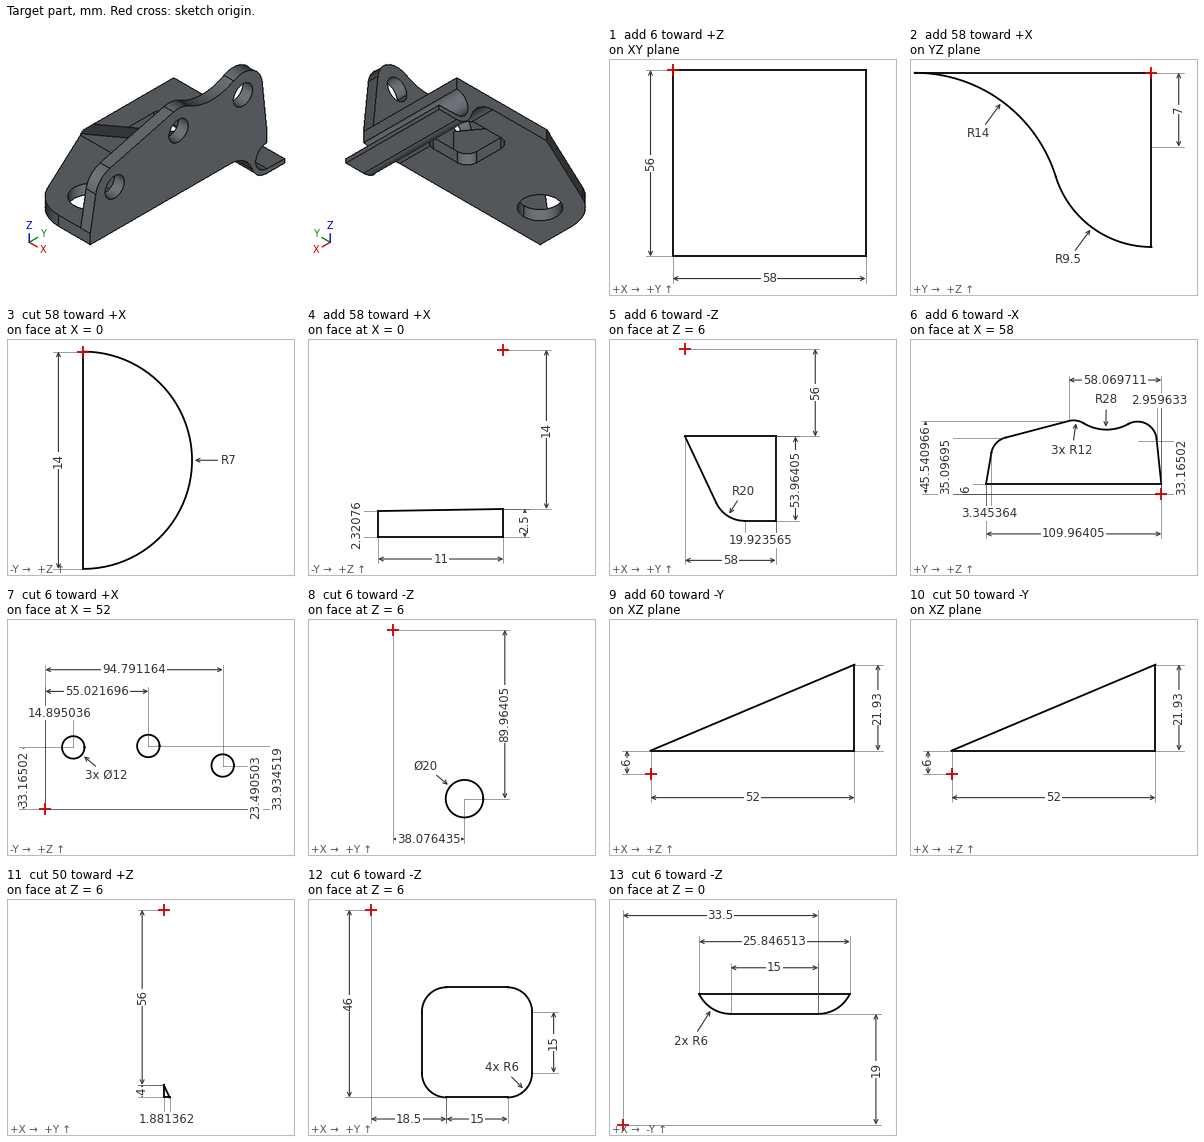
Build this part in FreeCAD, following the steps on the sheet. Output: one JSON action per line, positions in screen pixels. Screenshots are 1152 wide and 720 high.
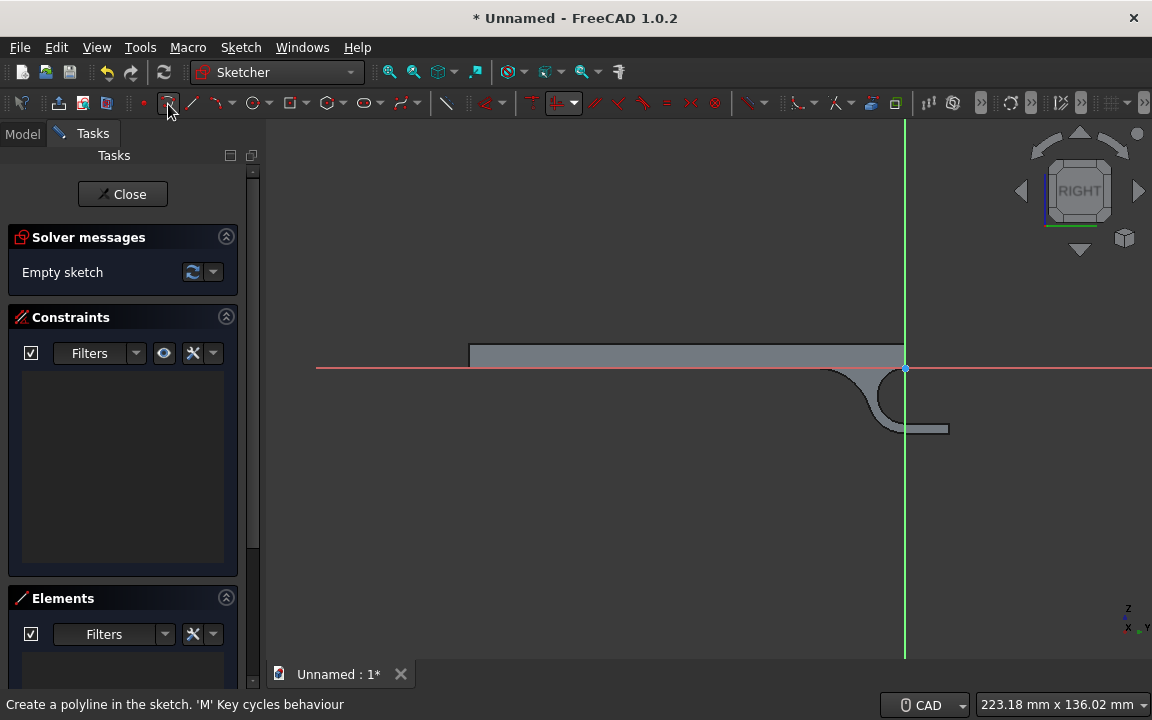
{"action": "left_click", "coordinate": [482, 267]}
{"action": "left_click", "coordinate": [469, 344]}
{"action": "left_click", "coordinate": [905, 344]}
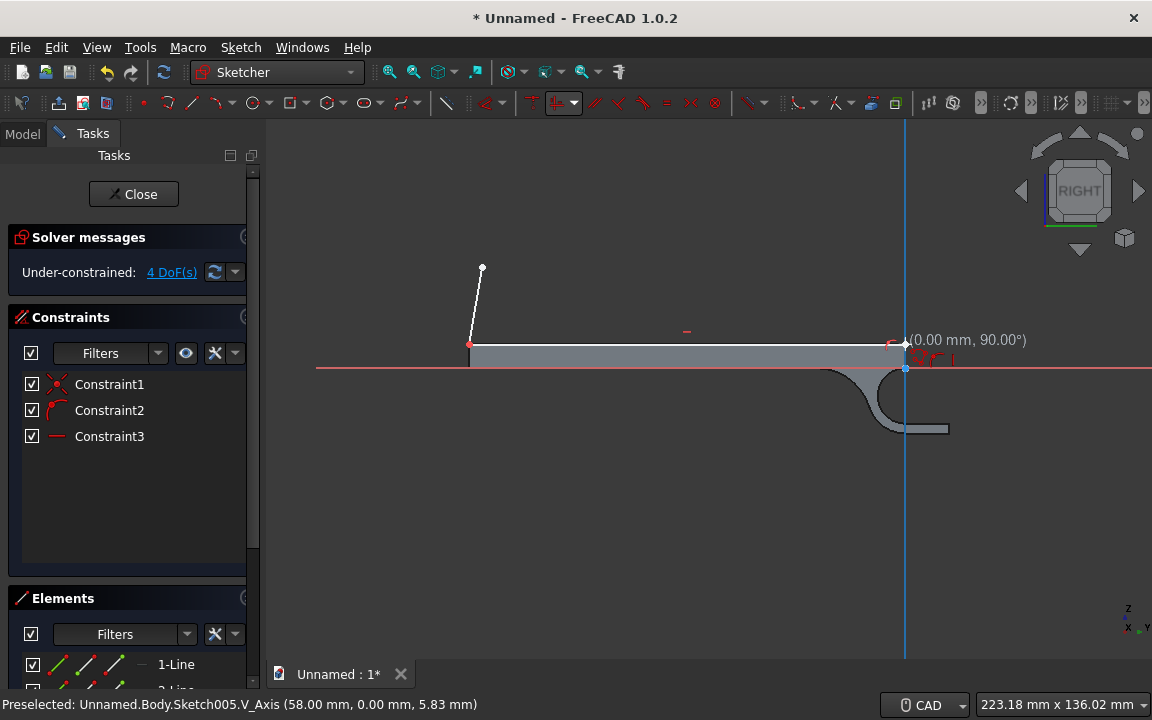
{"action": "scroll", "coordinate": [894, 232], "scroll_direction": "up", "scroll_amount": 2}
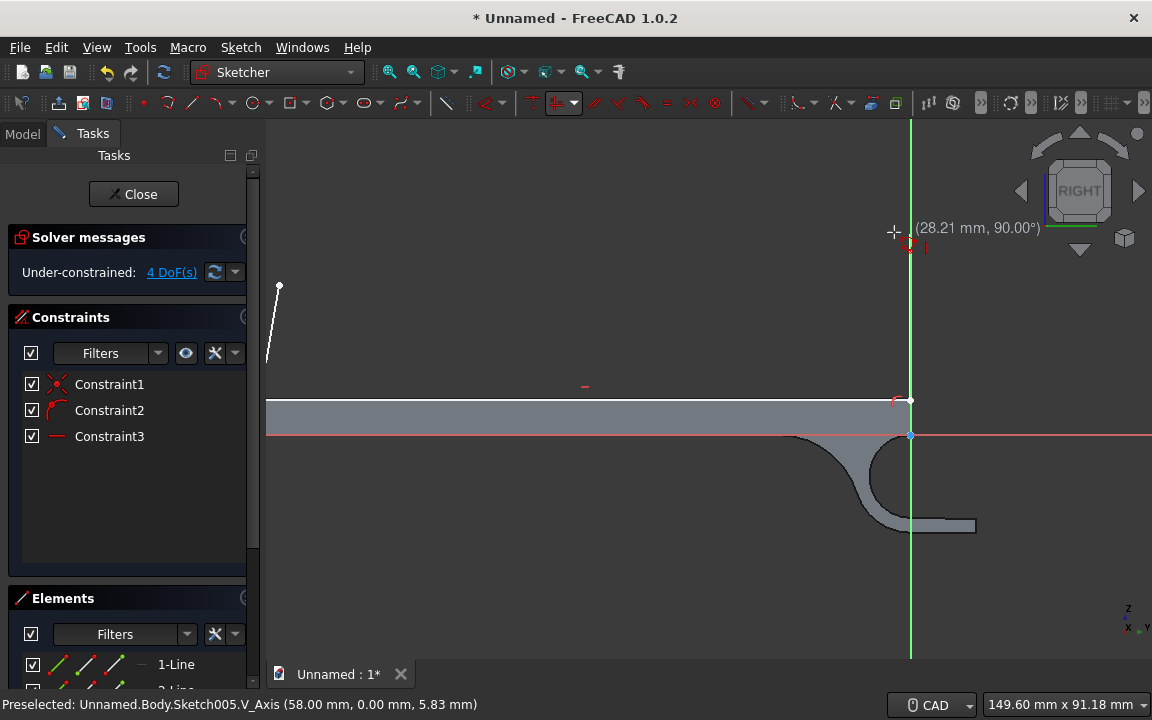
{"action": "left_click", "coordinate": [893, 231]}
{"action": "right_click", "coordinate": [893, 231]}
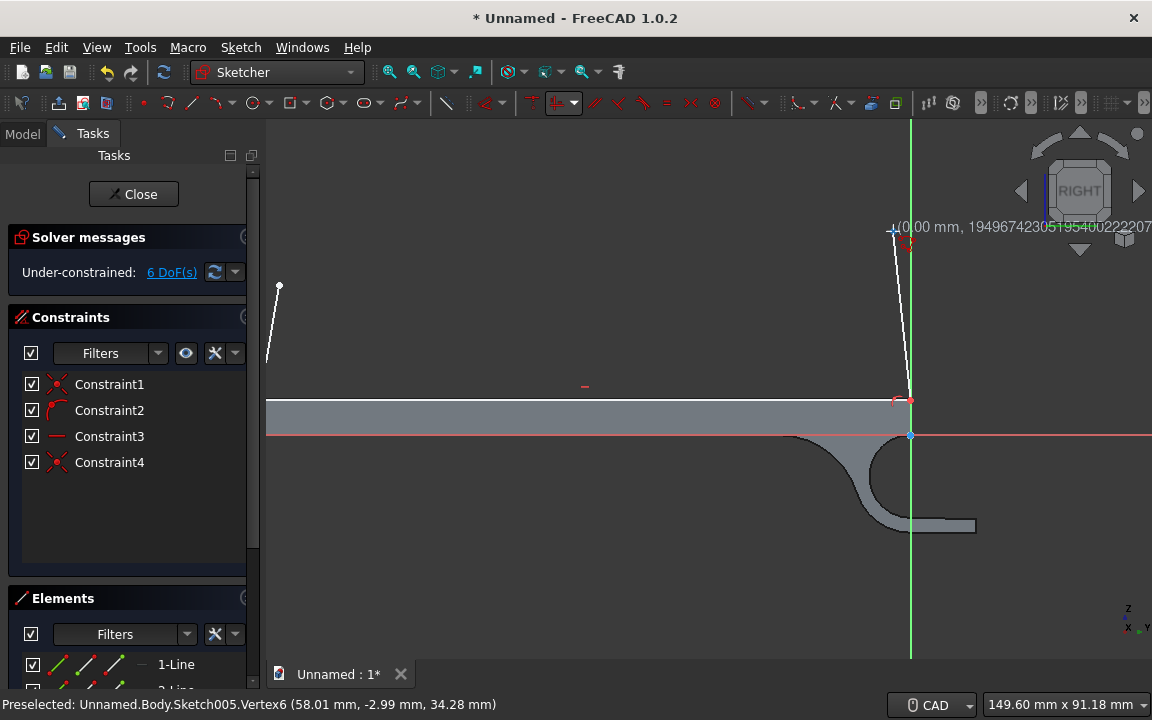
{"action": "key", "text": "g l"}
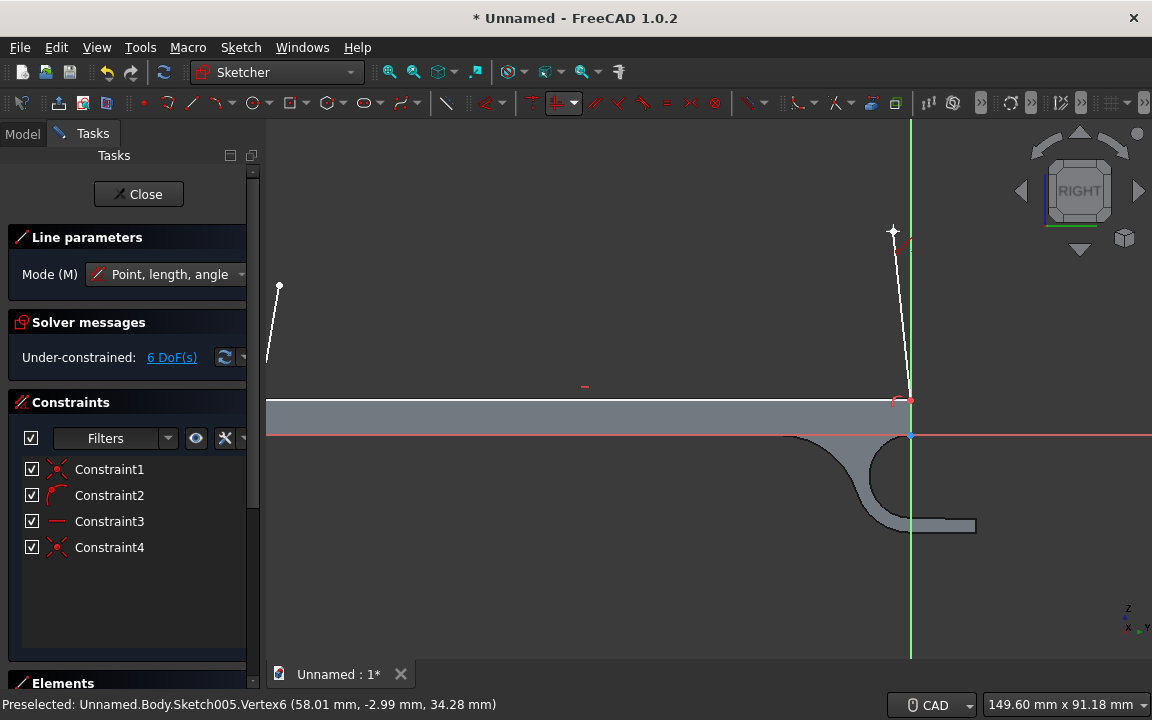
{"action": "left_click", "coordinate": [567, 165]}
{"action": "left_click", "coordinate": [331, 227]}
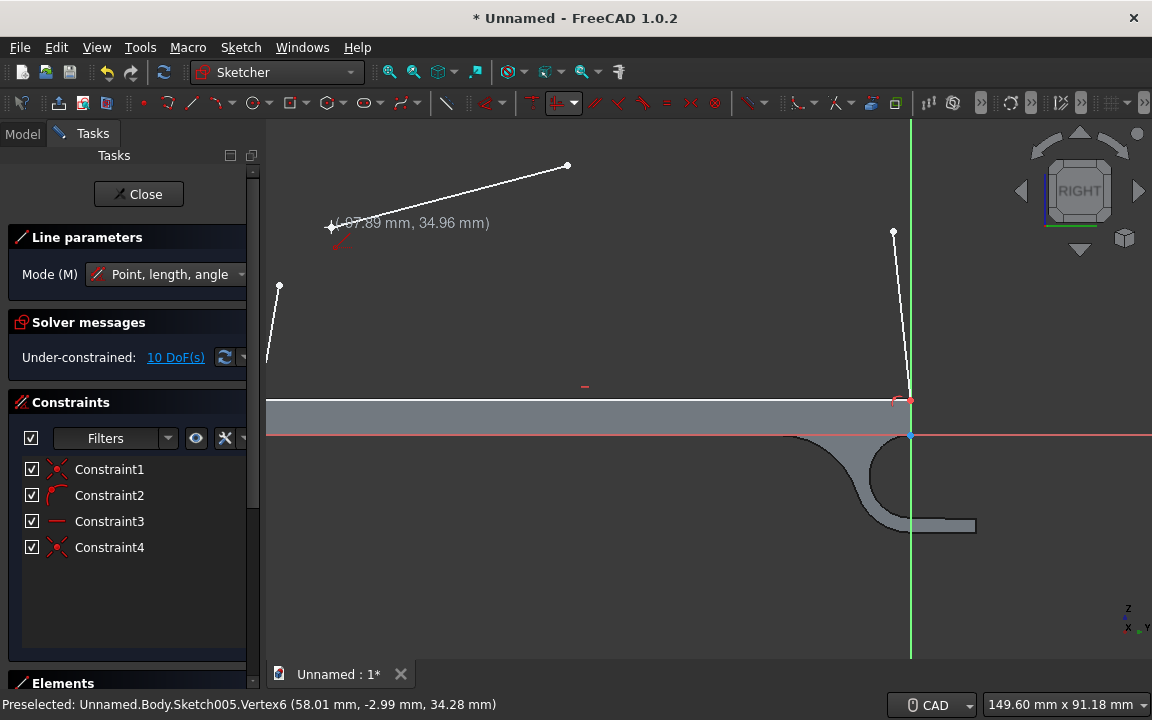
{"action": "left_click", "coordinate": [216, 104]}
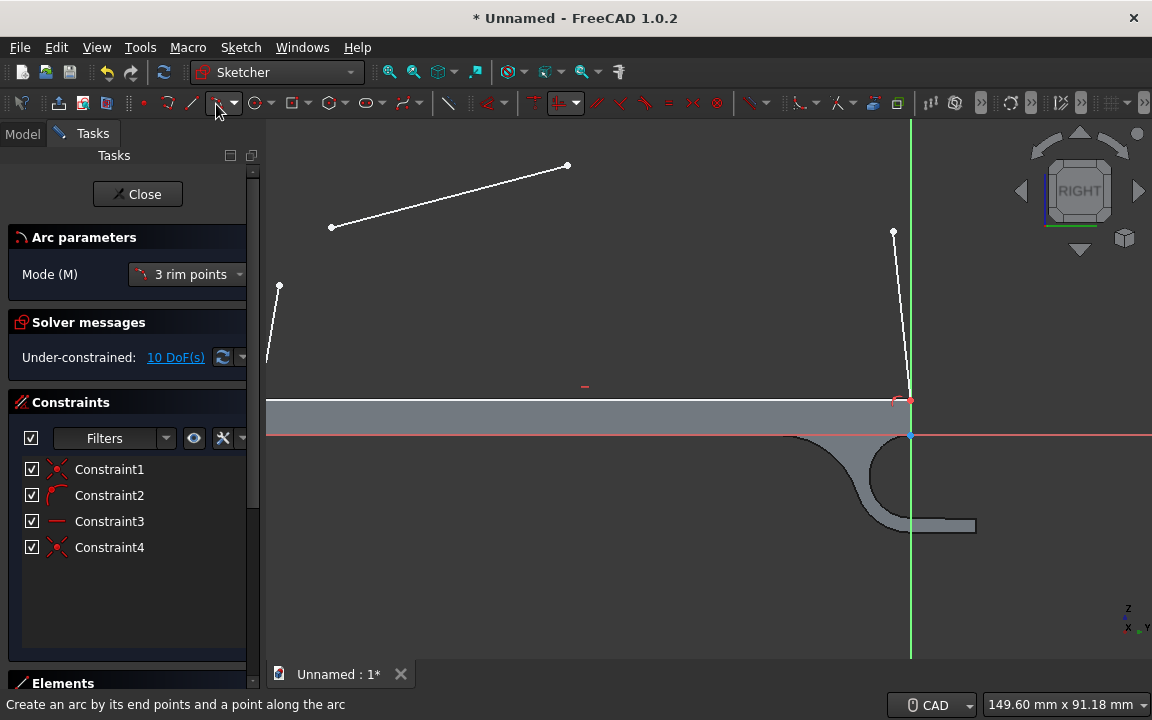
{"action": "left_click", "coordinate": [893, 232]}
{"action": "left_click", "coordinate": [788, 176]}
{"action": "left_click", "coordinate": [855, 176]}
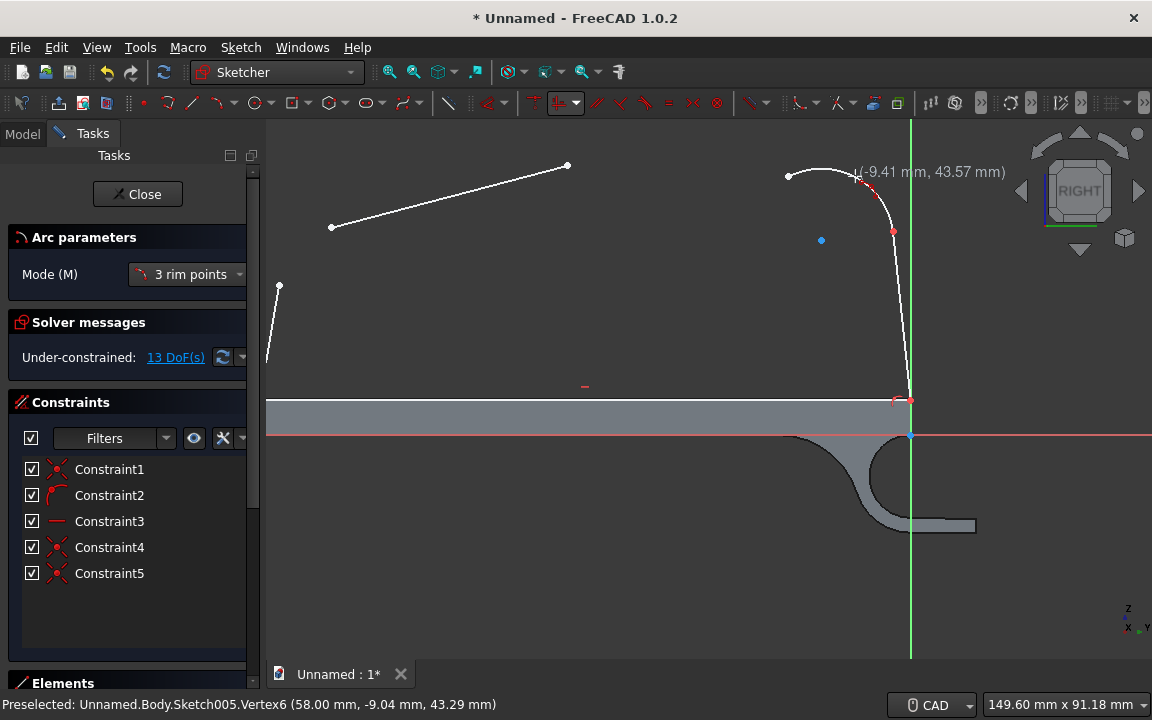
{"action": "left_click", "coordinate": [788, 177]}
{"action": "left_click", "coordinate": [622, 173]}
{"action": "left_click", "coordinate": [704, 197]}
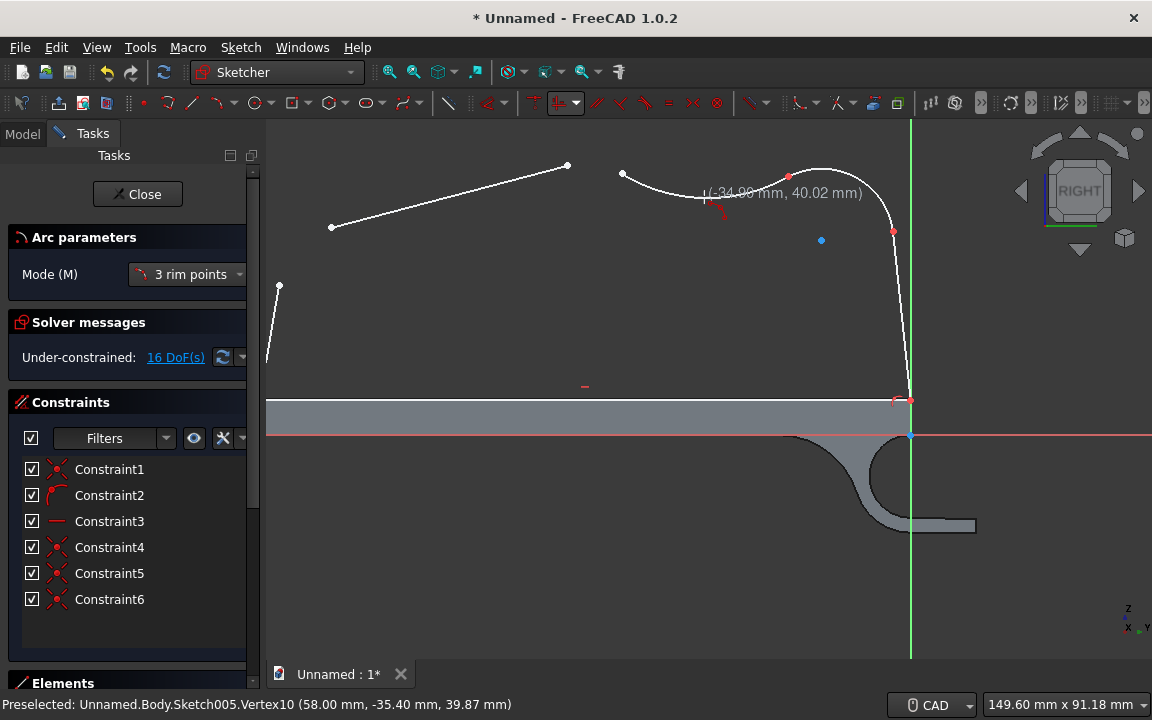
{"action": "left_click", "coordinate": [622, 174]}
{"action": "left_click", "coordinate": [567, 166]}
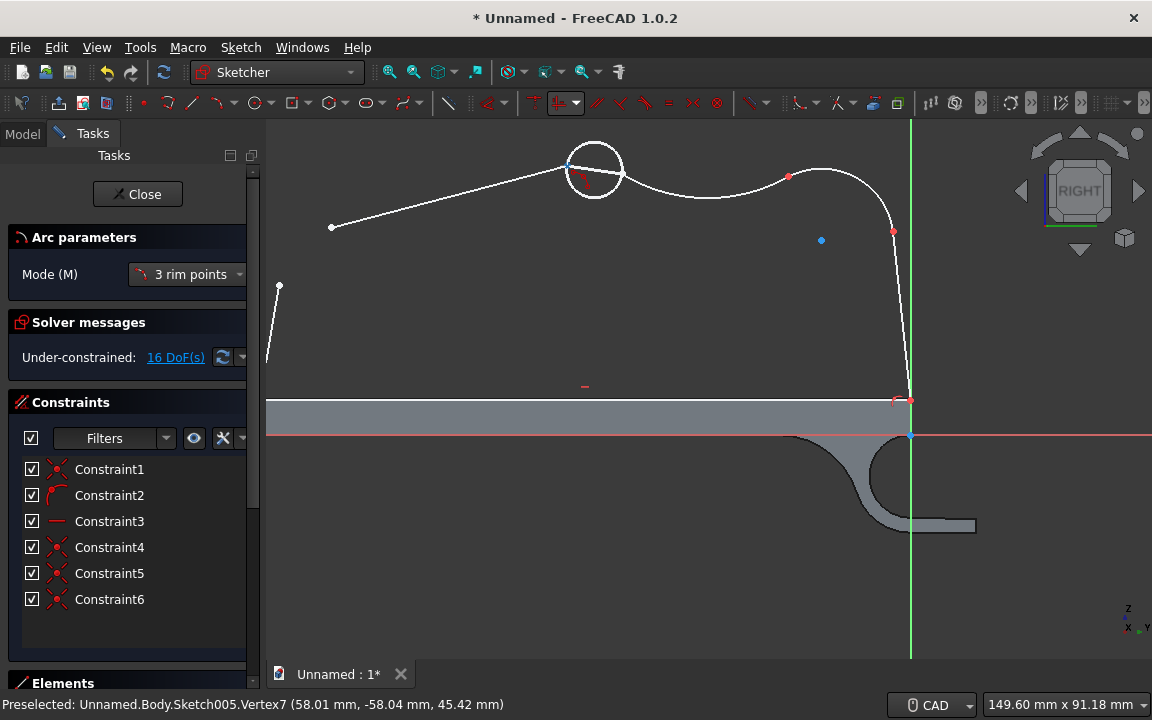
{"action": "scroll", "coordinate": [595, 164], "scroll_direction": "up", "scroll_amount": 6}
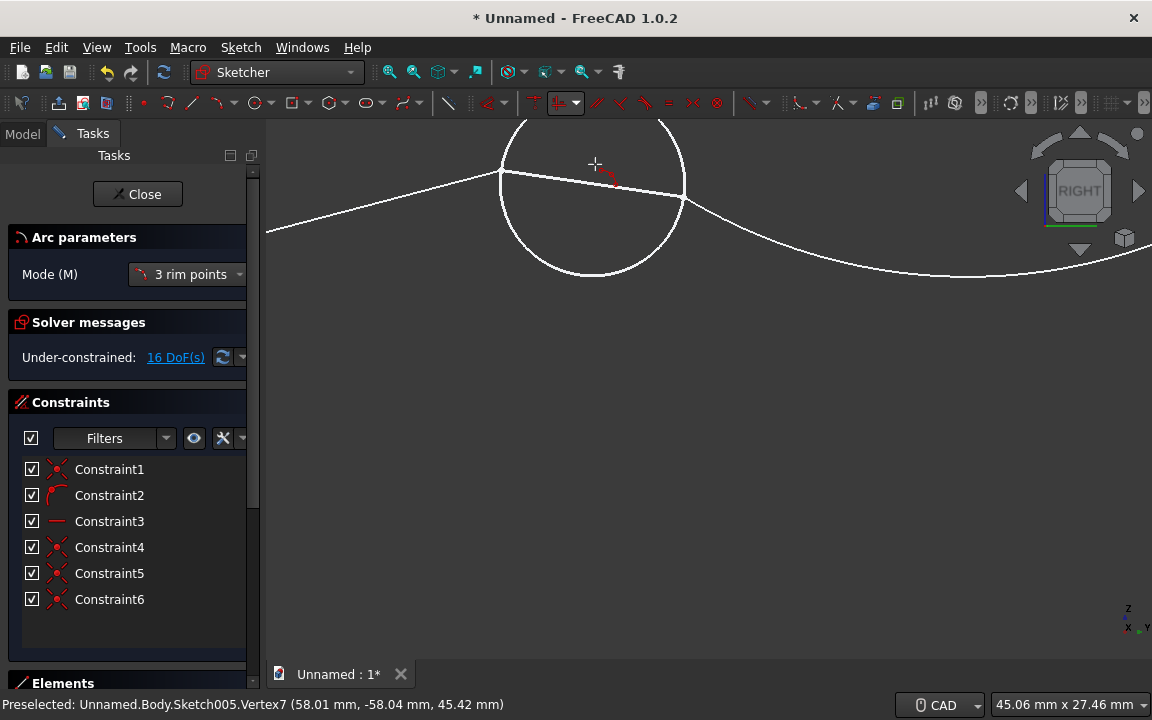
{"action": "left_click", "coordinate": [594, 163]}